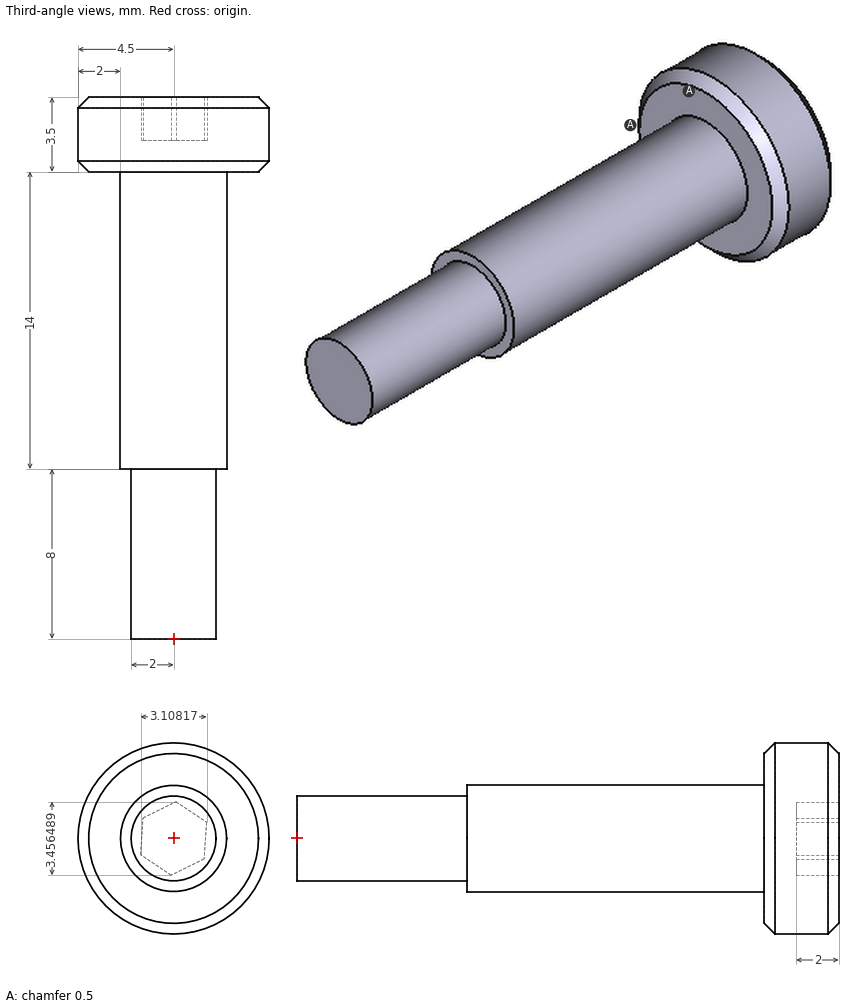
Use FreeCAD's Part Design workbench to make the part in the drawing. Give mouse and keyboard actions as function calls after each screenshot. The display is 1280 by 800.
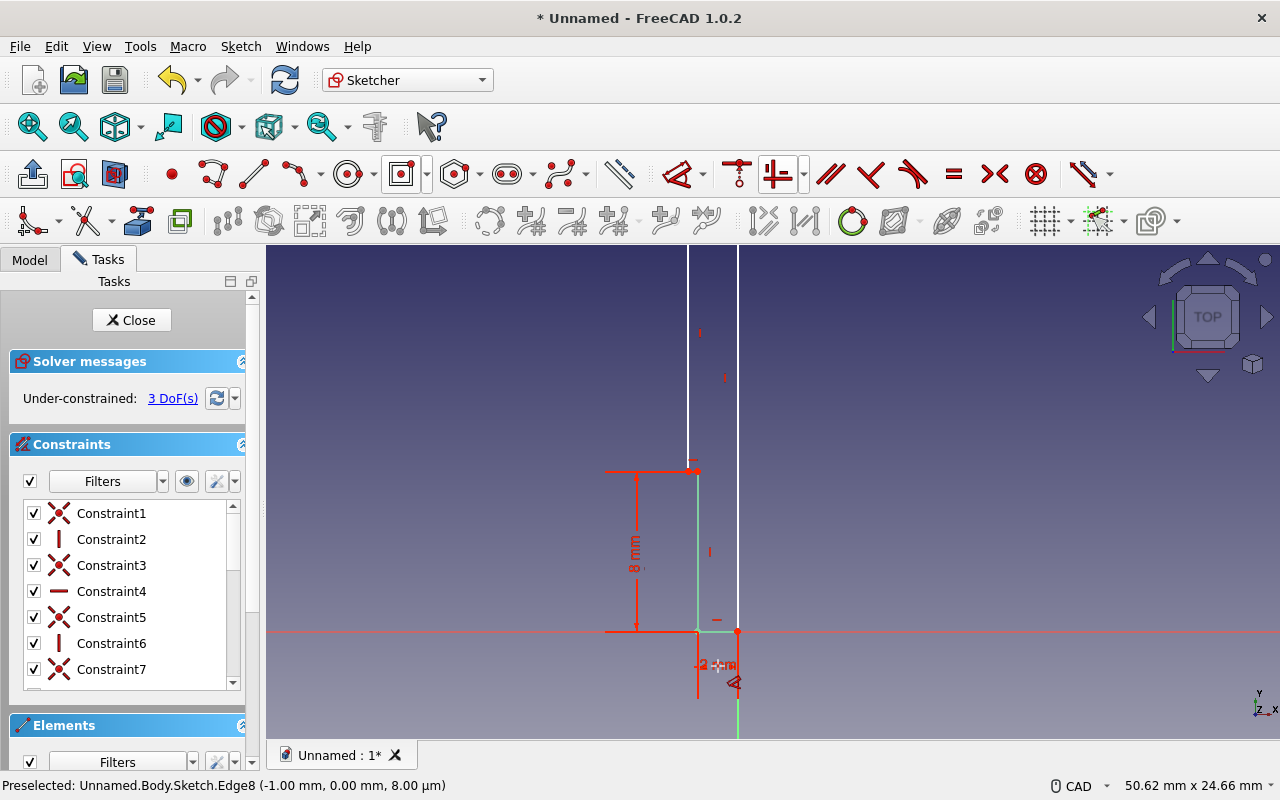
click(688, 277)
click(654, 372)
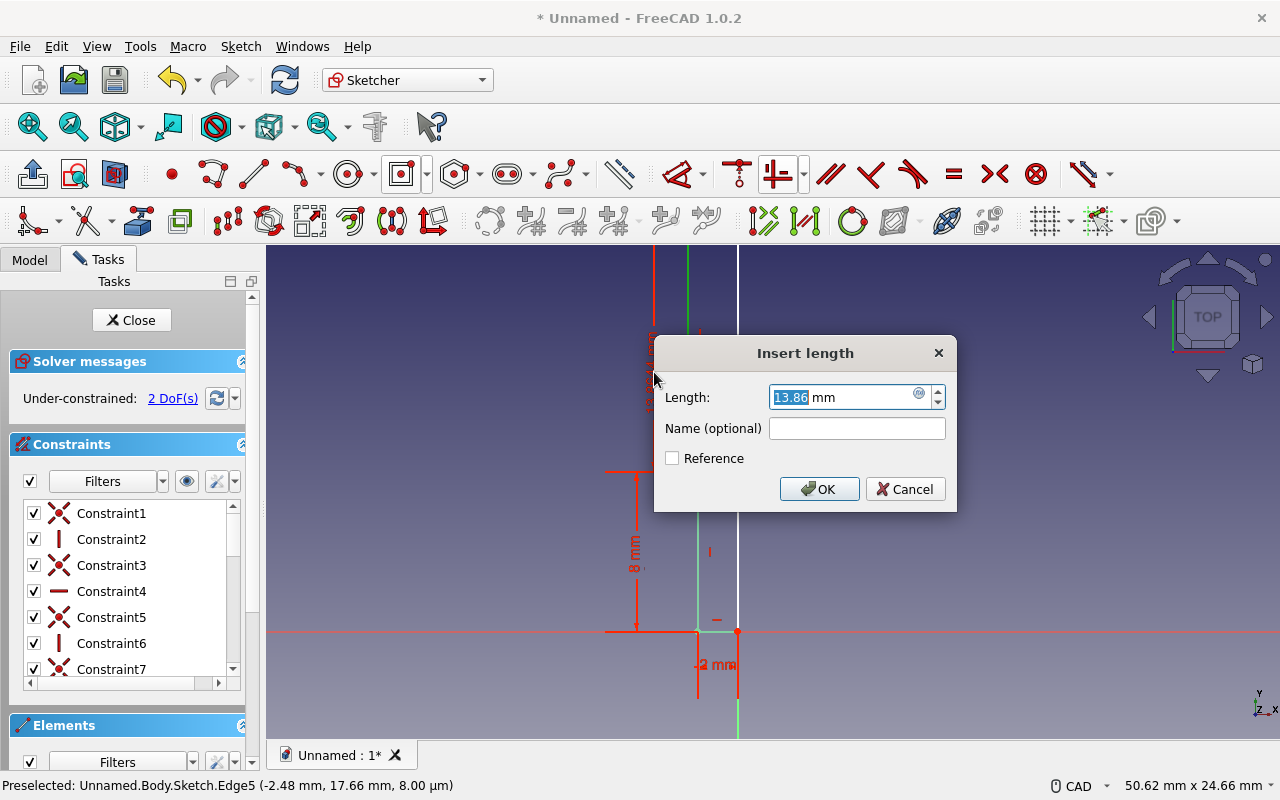
text(14)
key(Return)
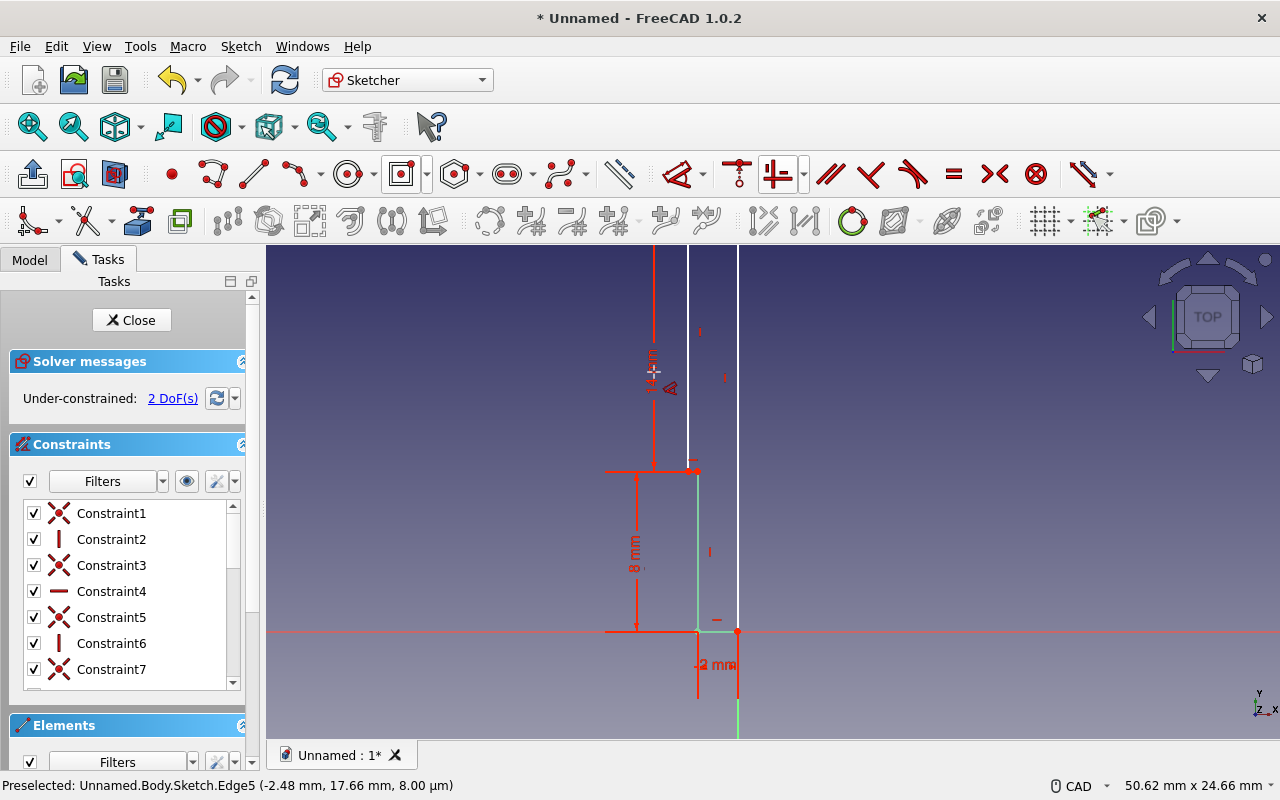
scroll(719, 633, down, 3)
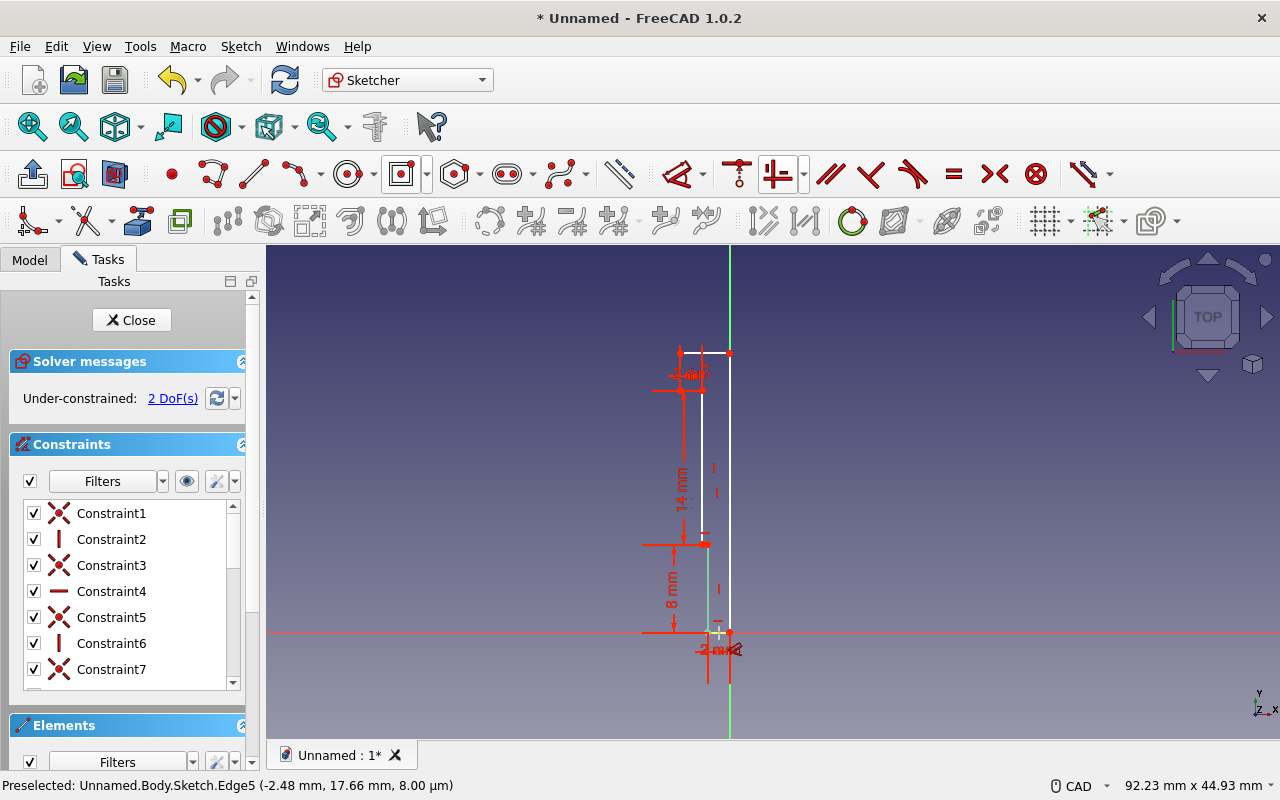
click(715, 353)
click(705, 319)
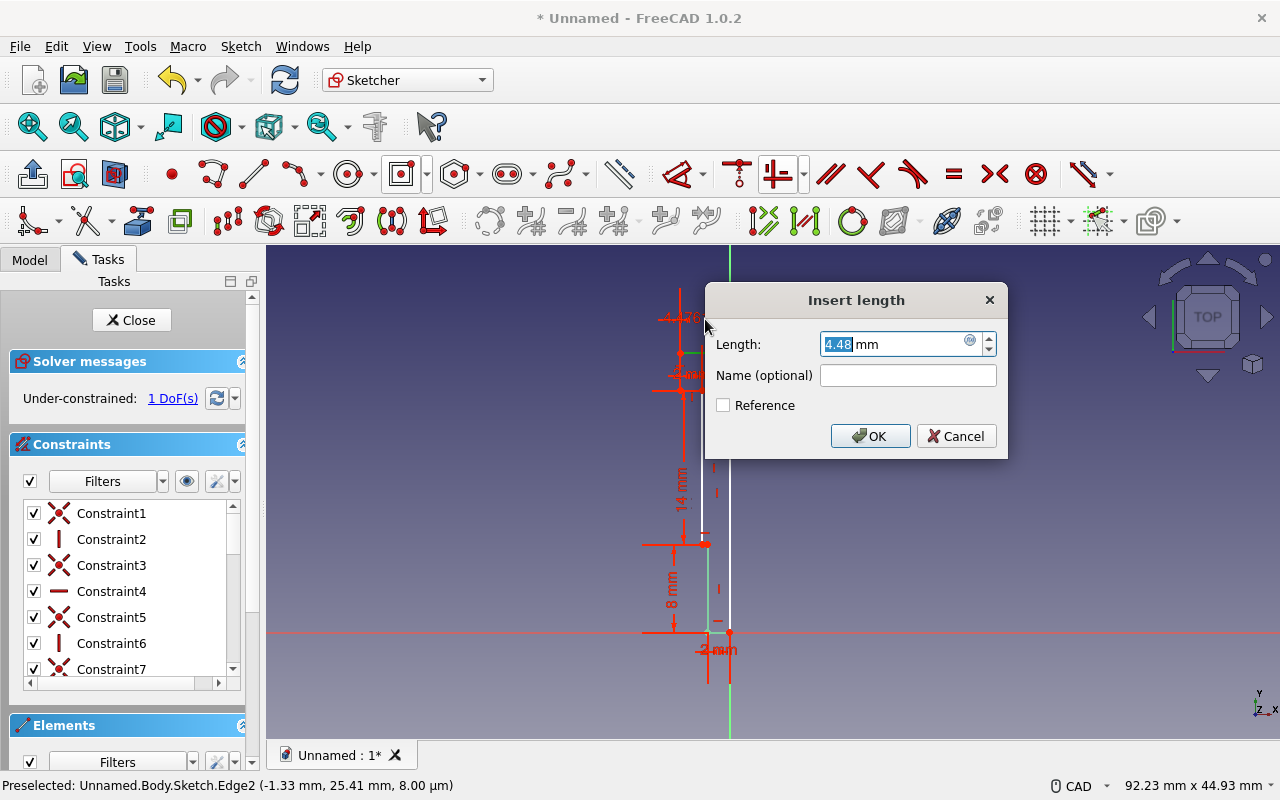
text(4.5)
key(Return)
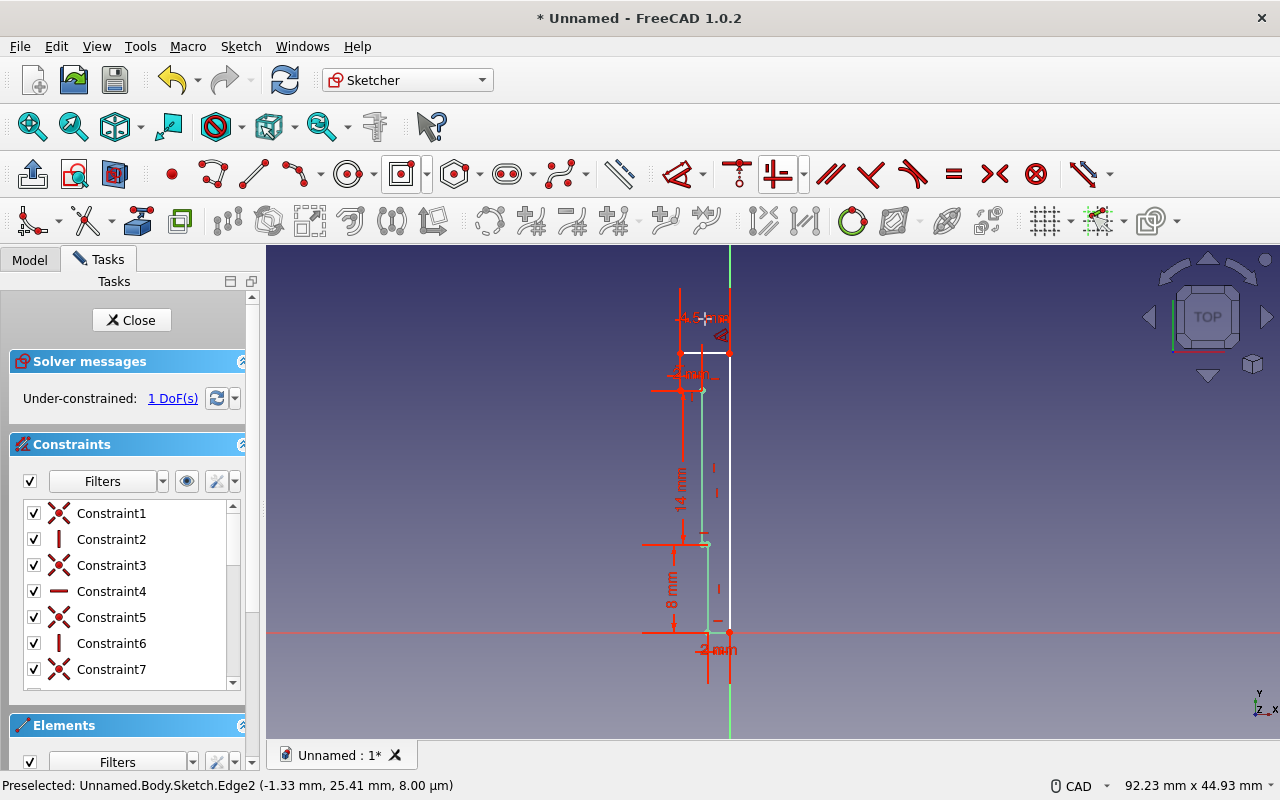
scroll(680, 365, up, 2)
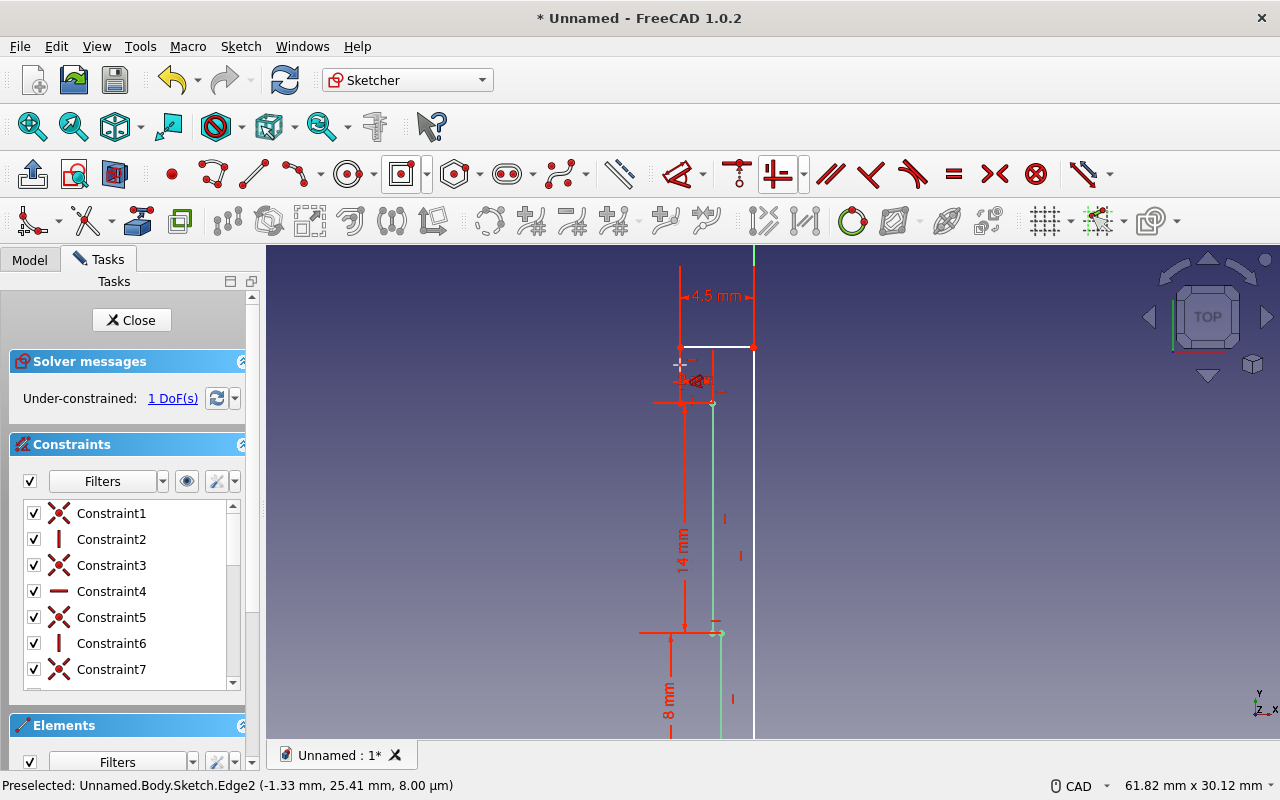
click(680, 364)
click(646, 363)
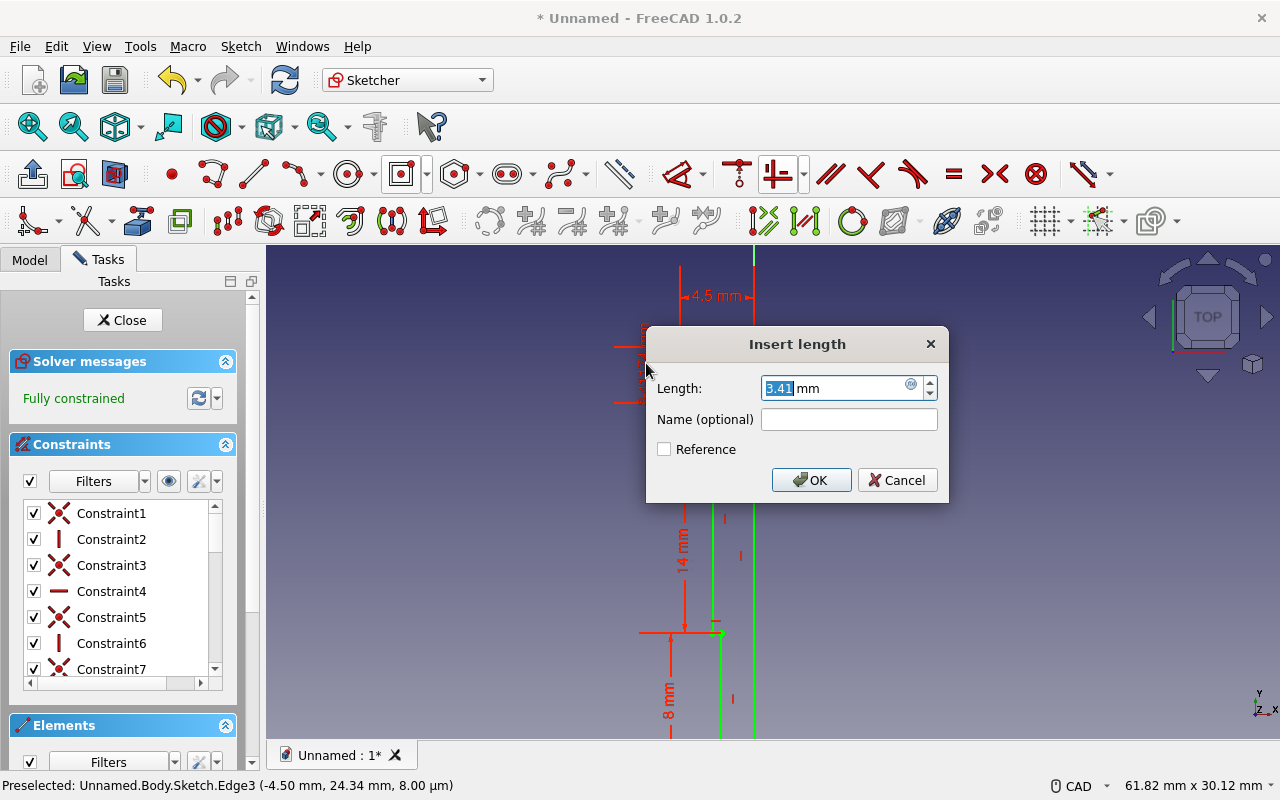
text(3.5)
key(Return)
key(Escape)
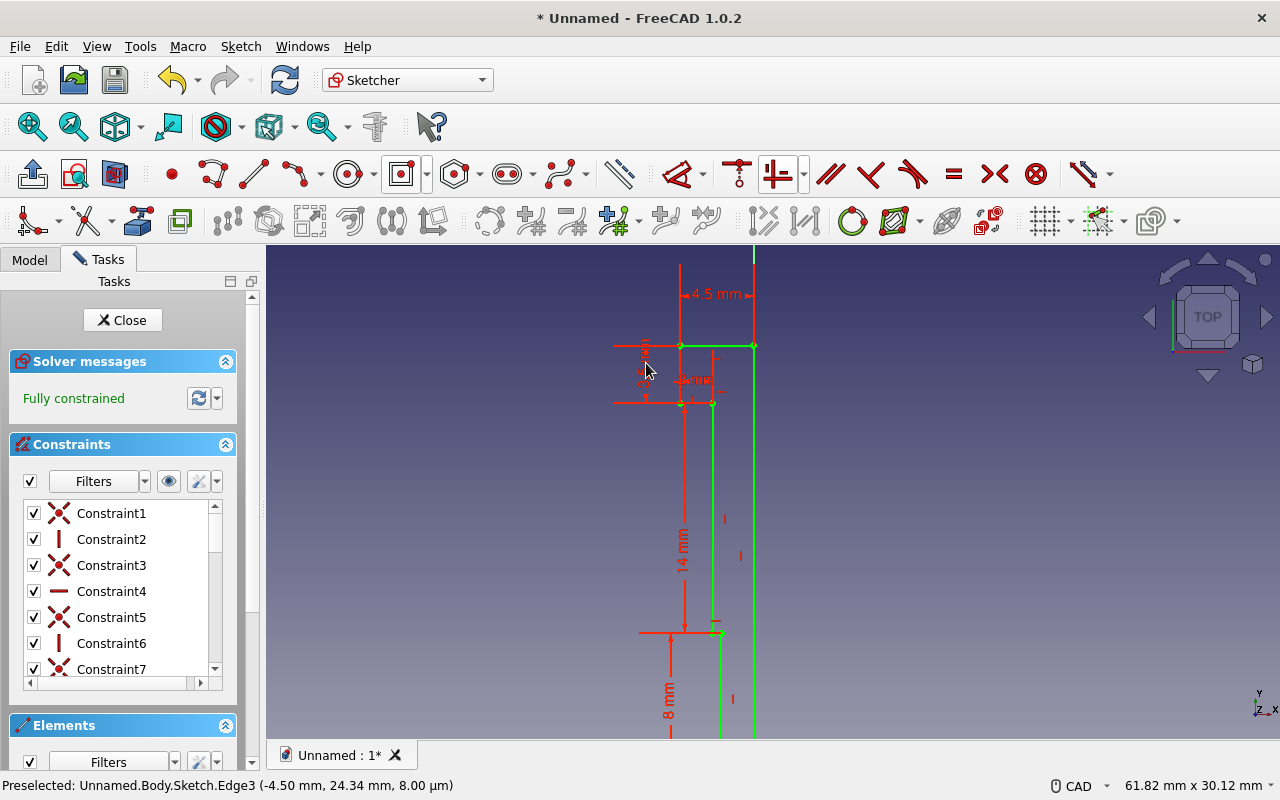
click(123, 320)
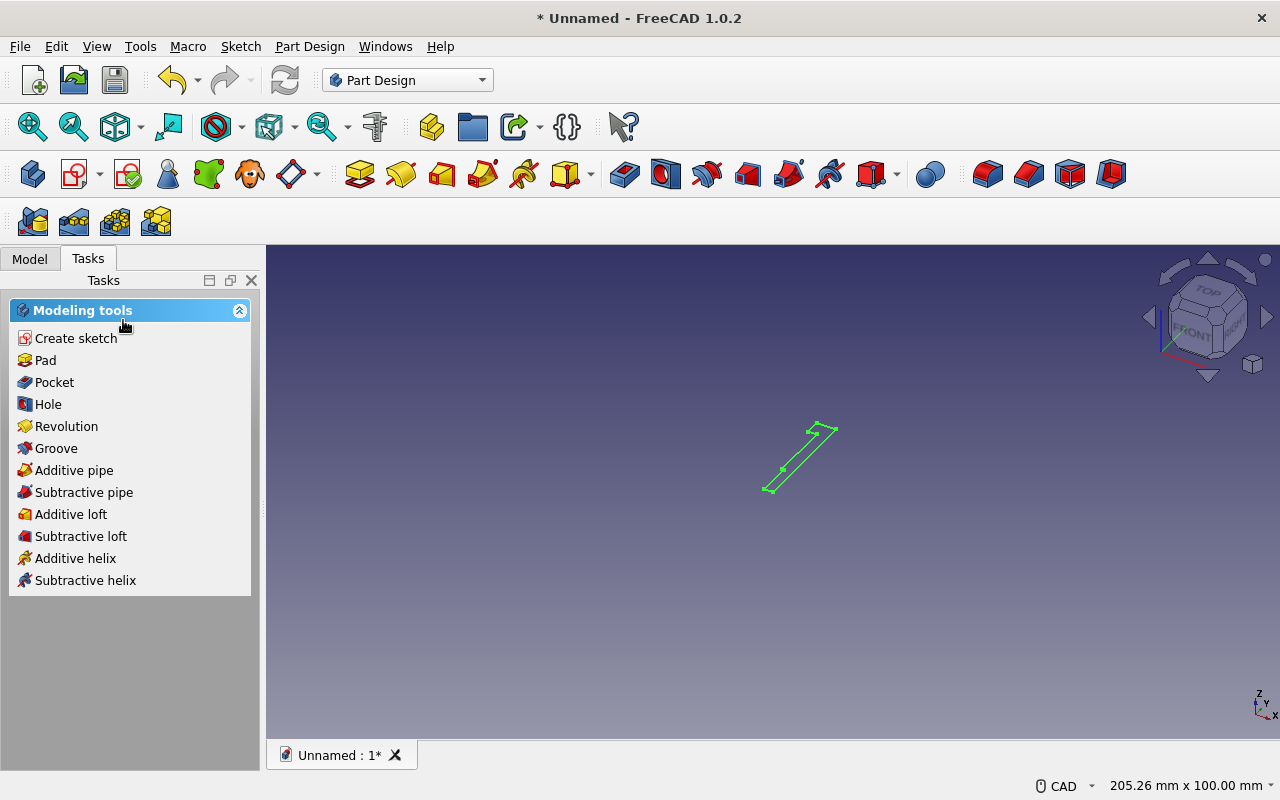
click(401, 174)